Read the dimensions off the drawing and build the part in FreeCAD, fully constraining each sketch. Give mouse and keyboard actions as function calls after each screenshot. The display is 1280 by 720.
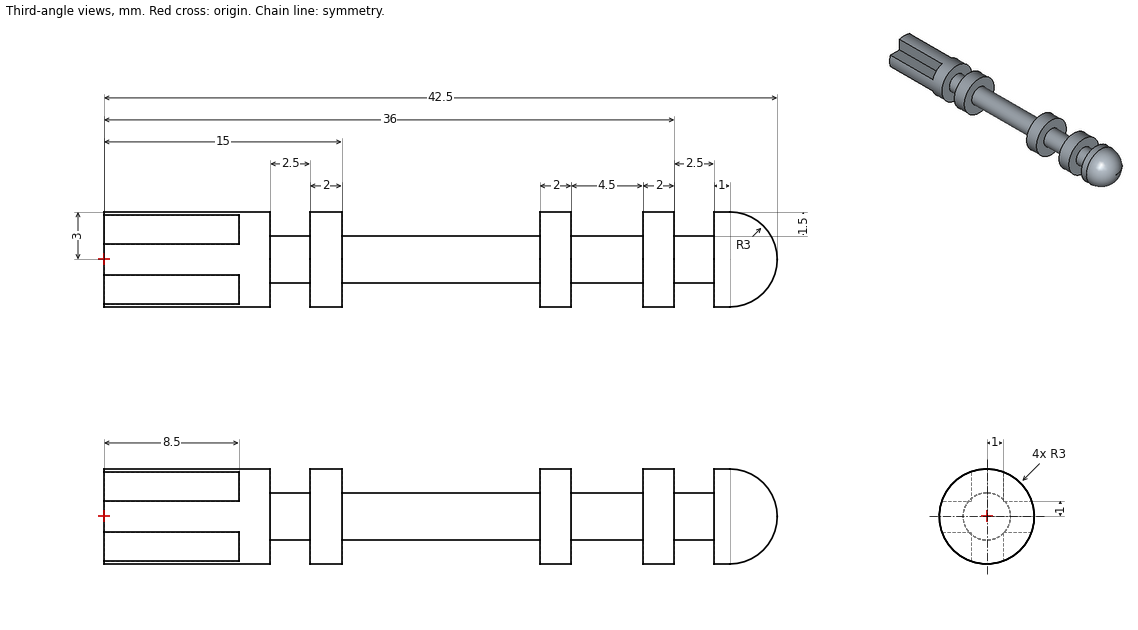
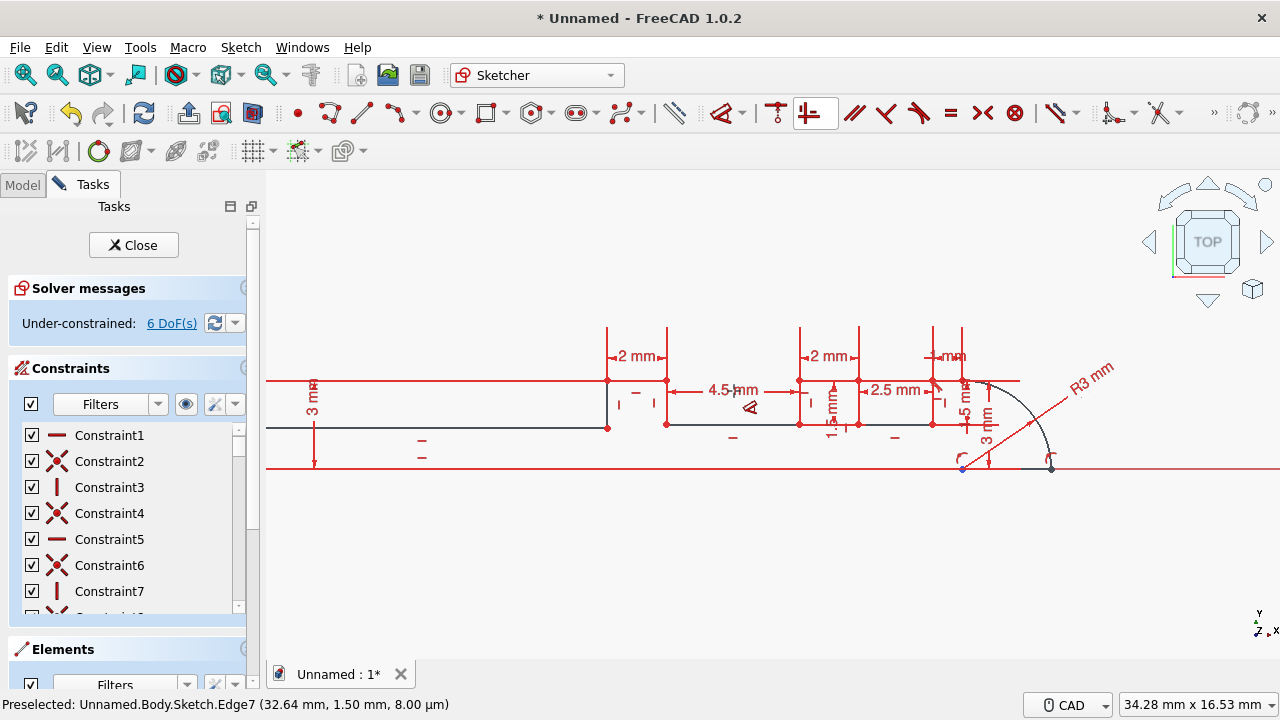
click(607, 395)
click(641, 404)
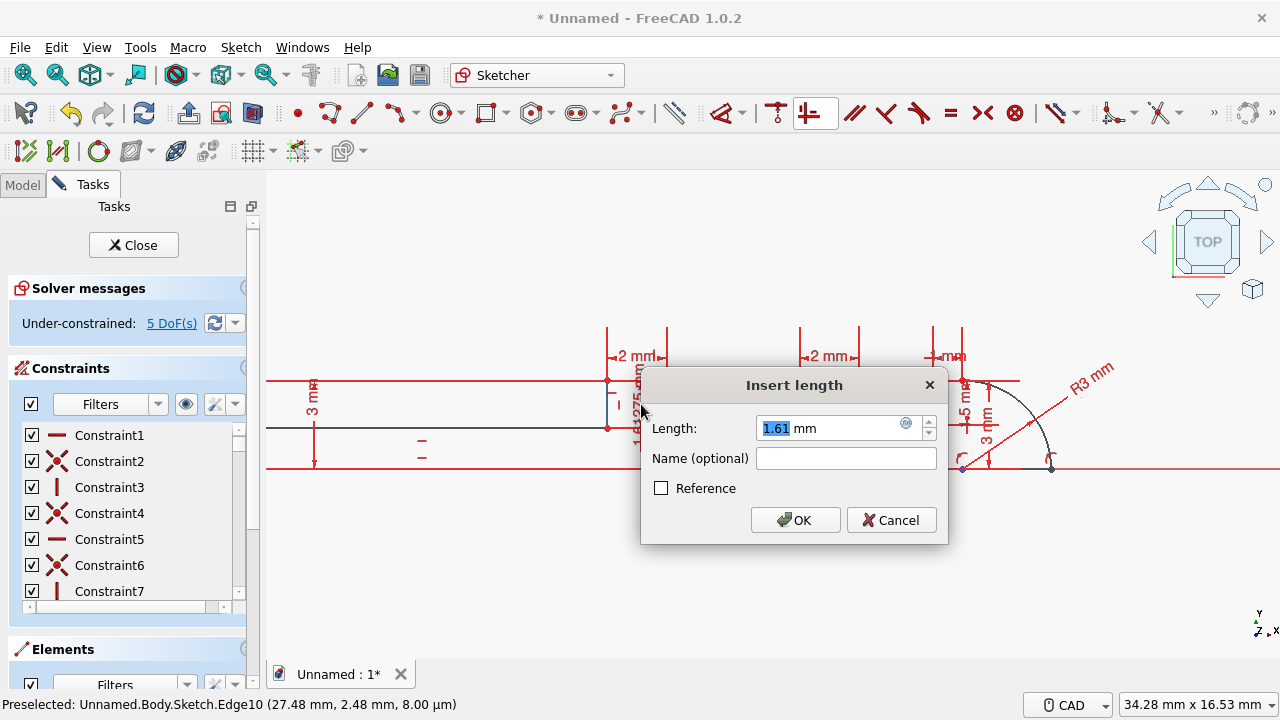
text(1.5)
key(Return)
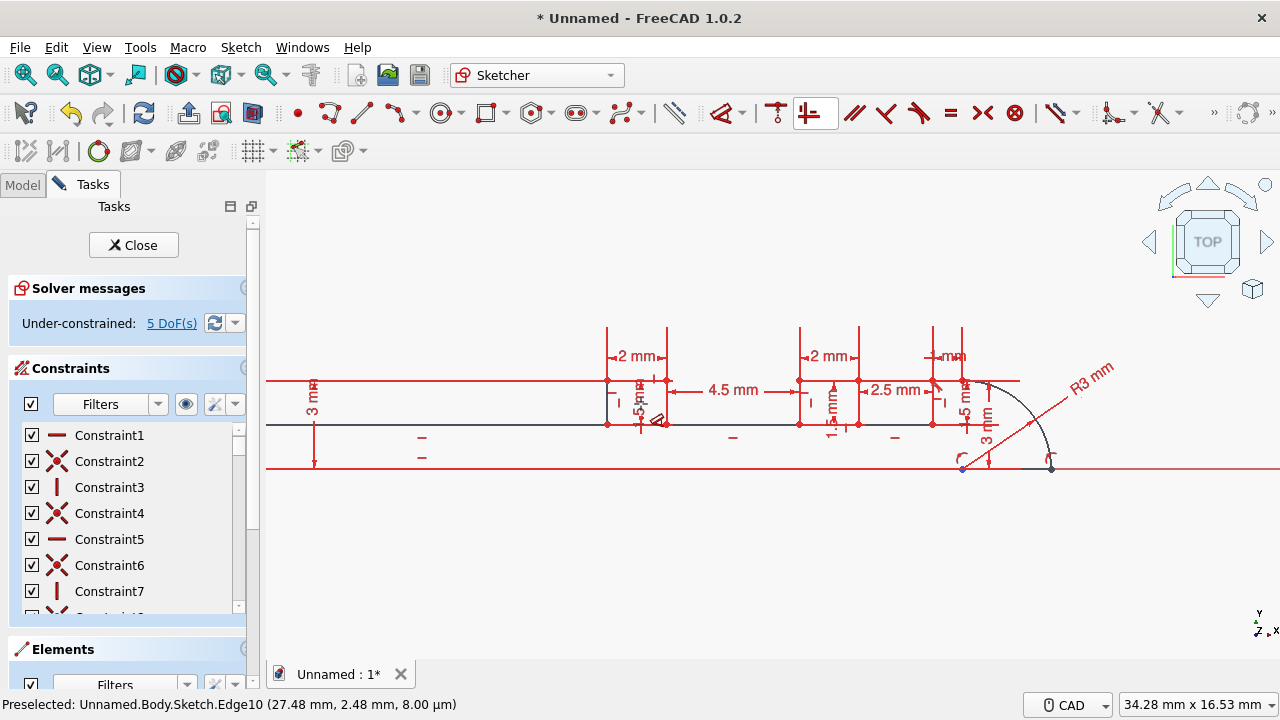
scroll(934, 406, down, 4)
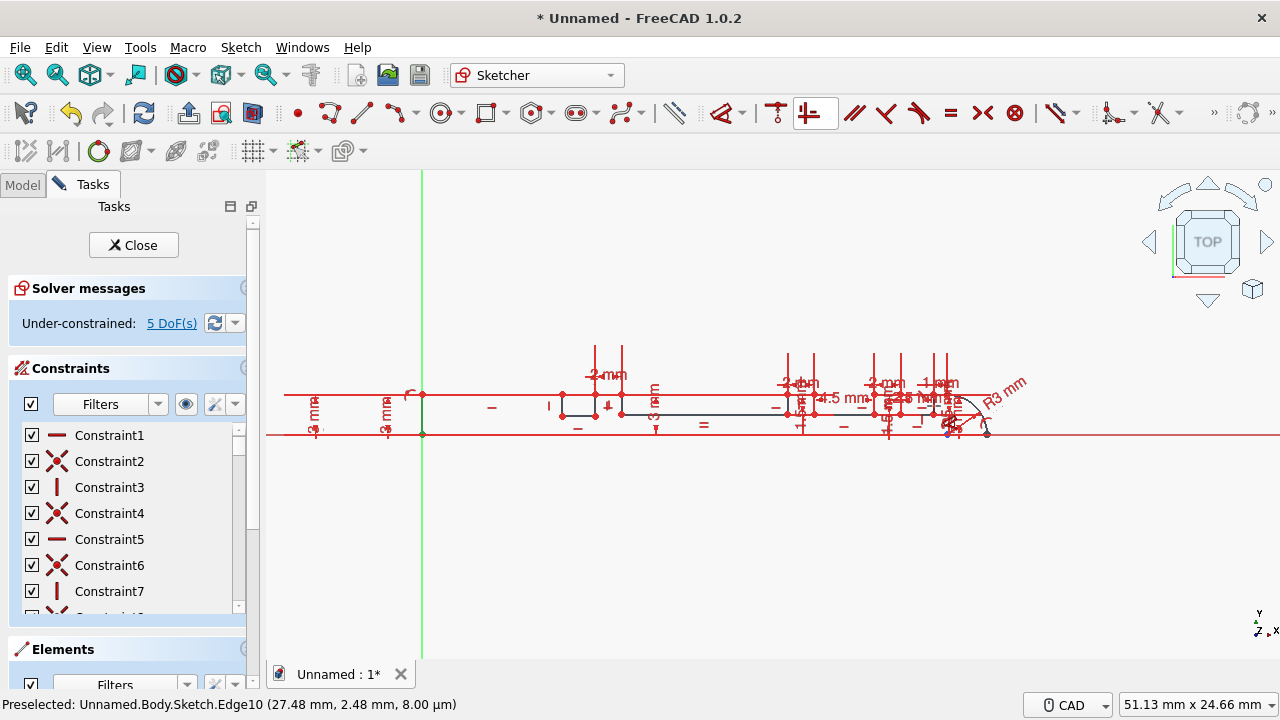
scroll(595, 401, up, 4)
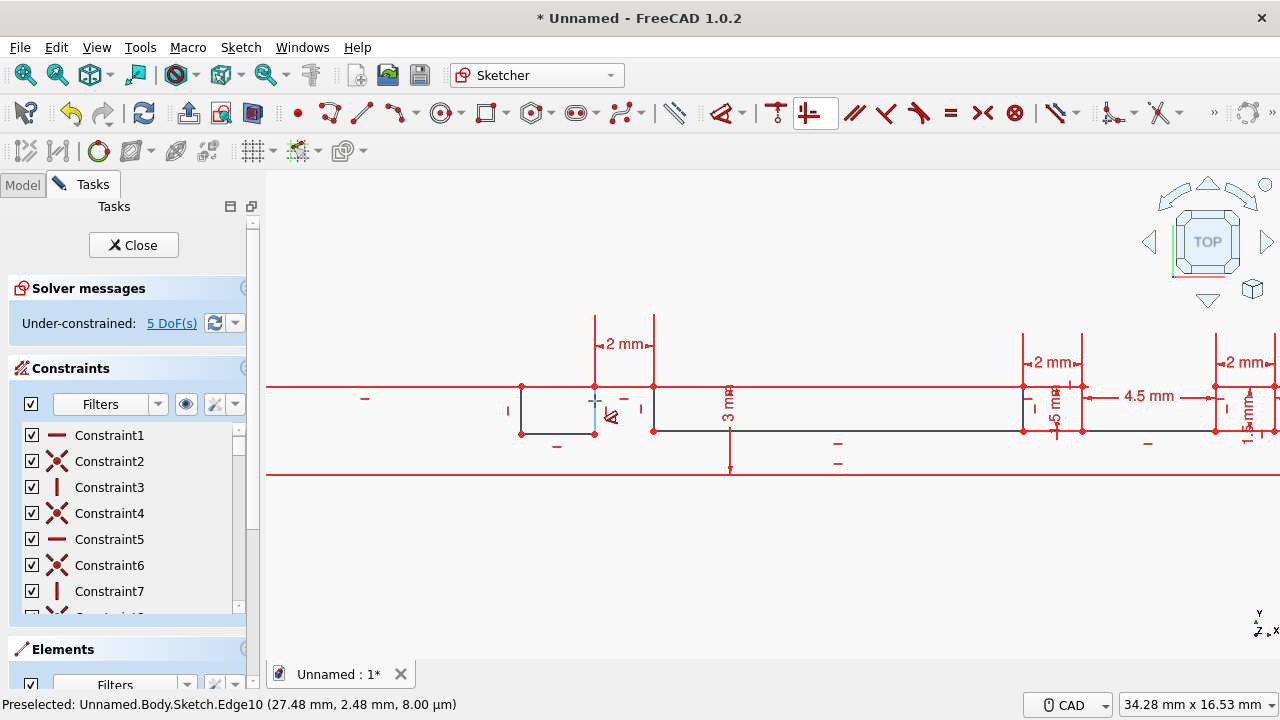
click(595, 401)
click(561, 411)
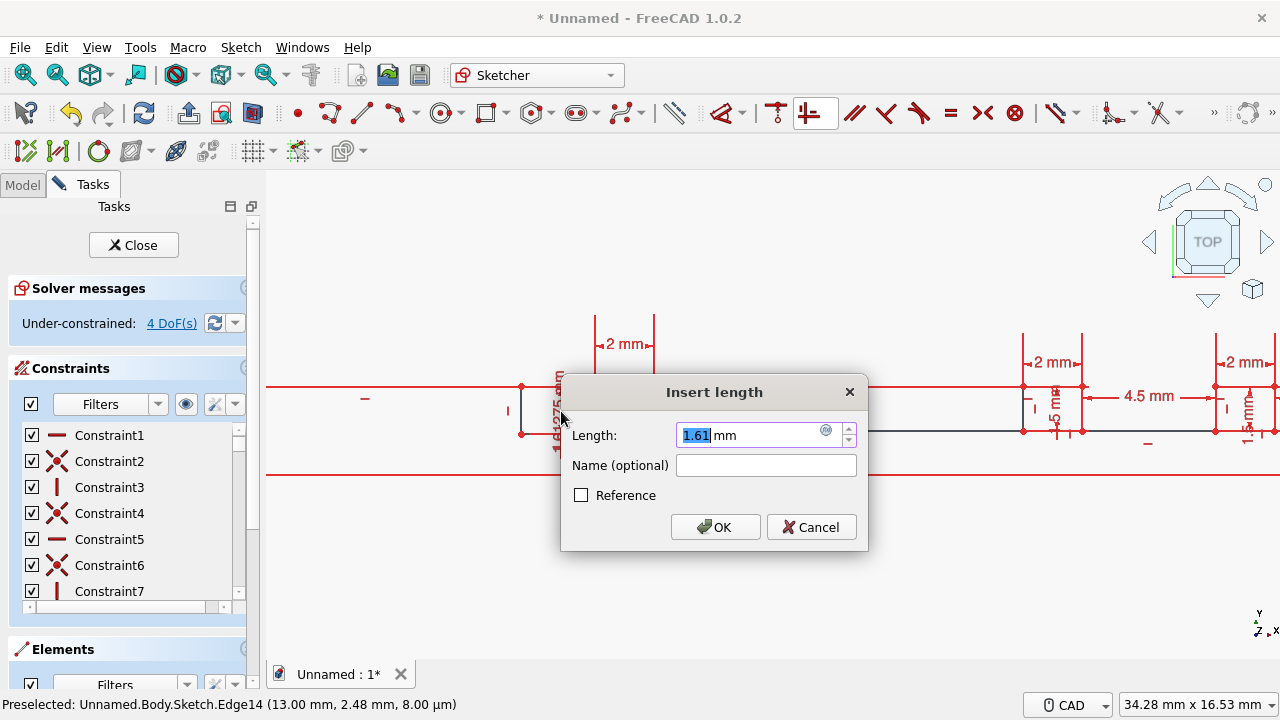
text(1.5)
key(Return)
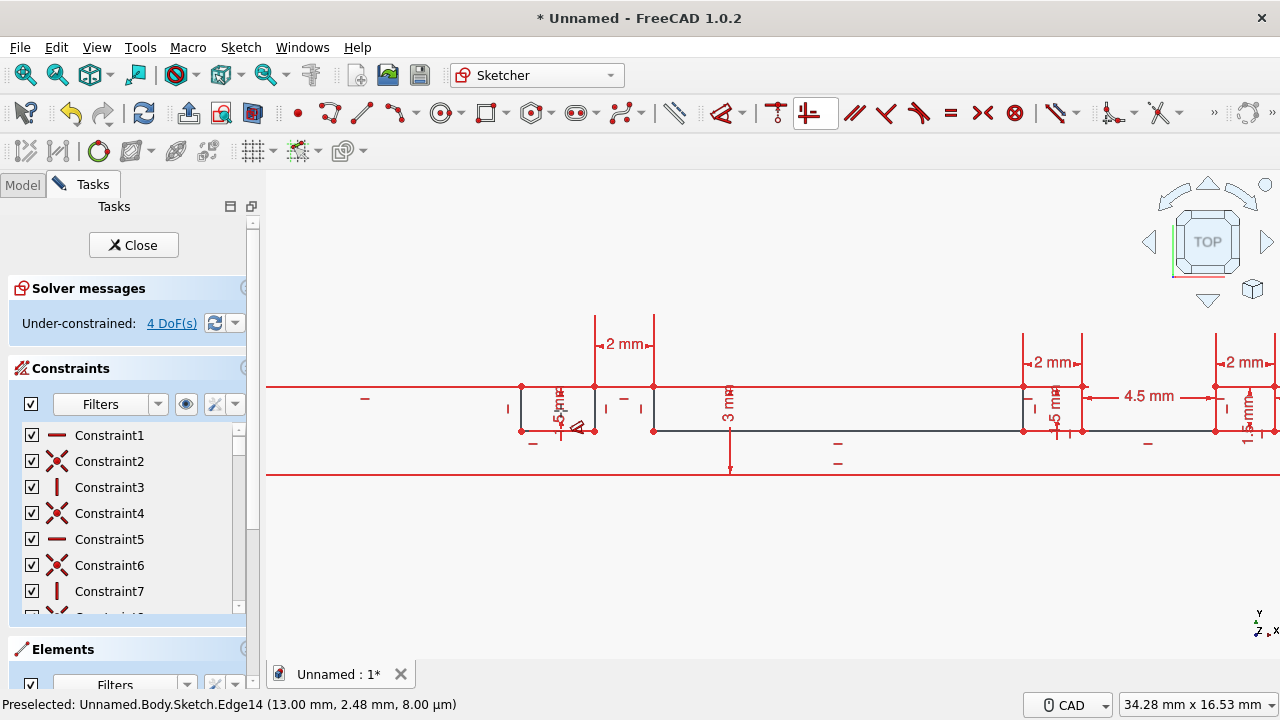
click(573, 431)
click(558, 489)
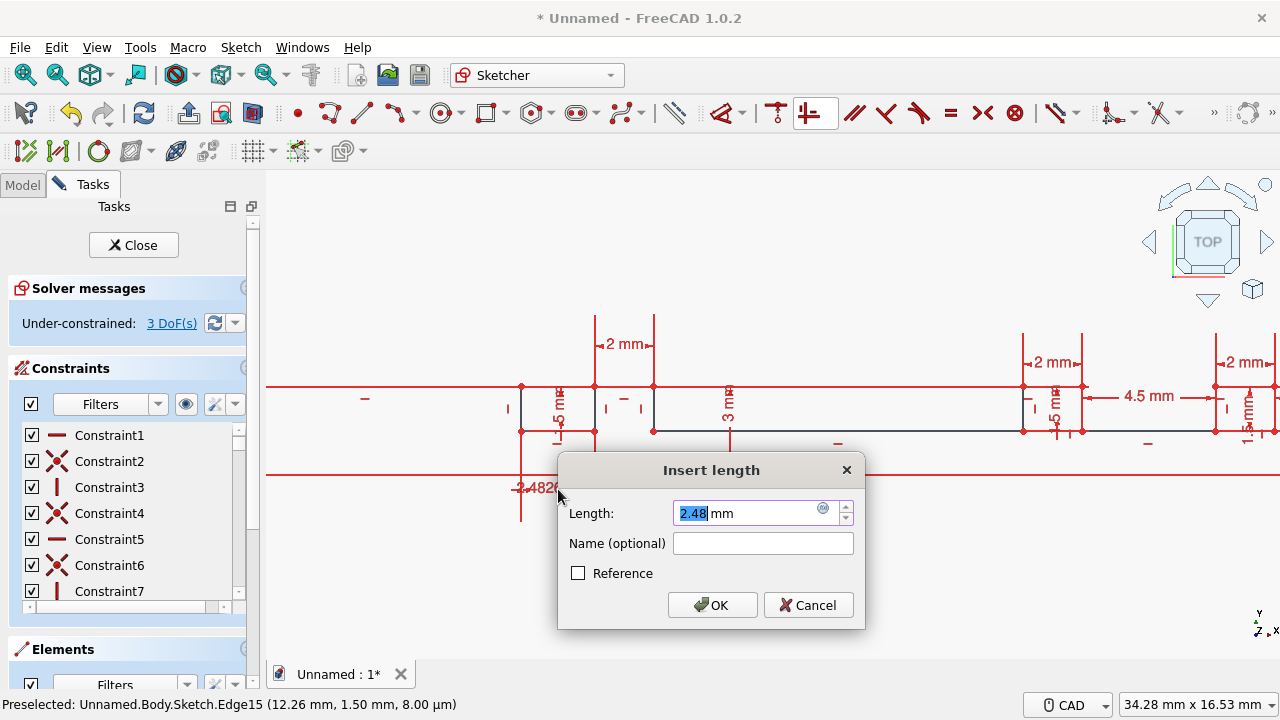
text(2.5)
key(Return)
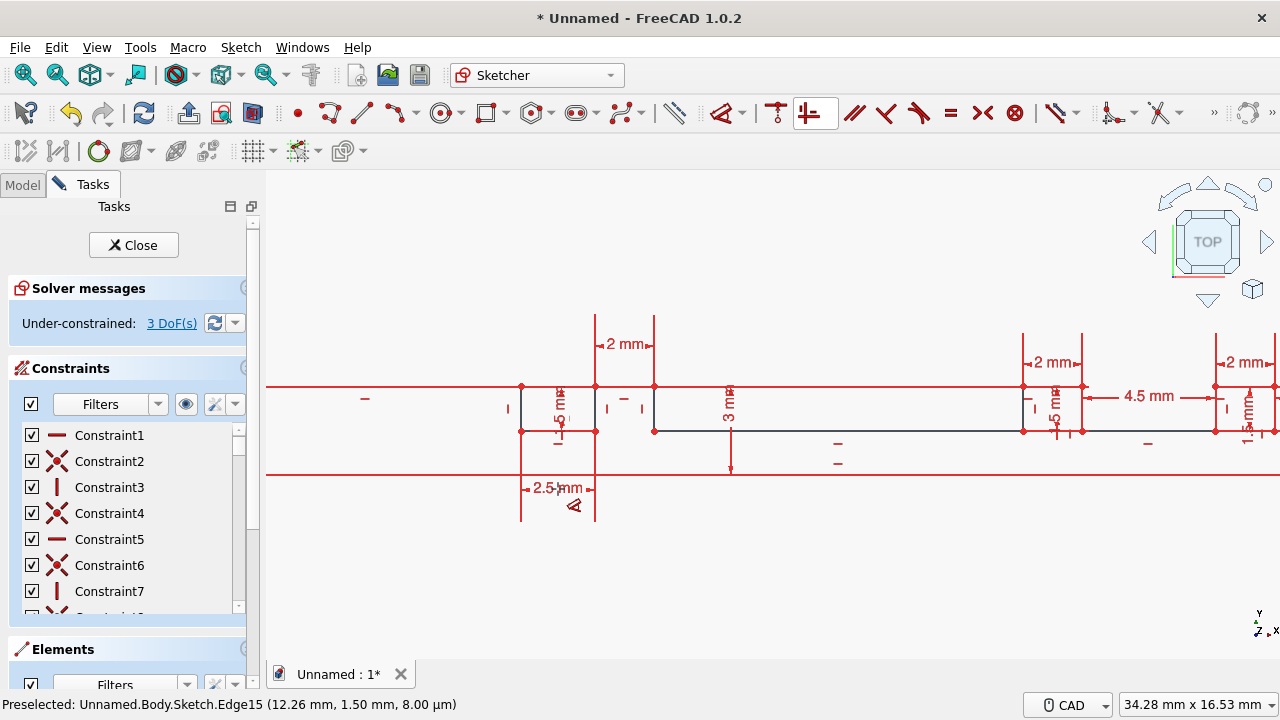
scroll(595, 401, down, 4)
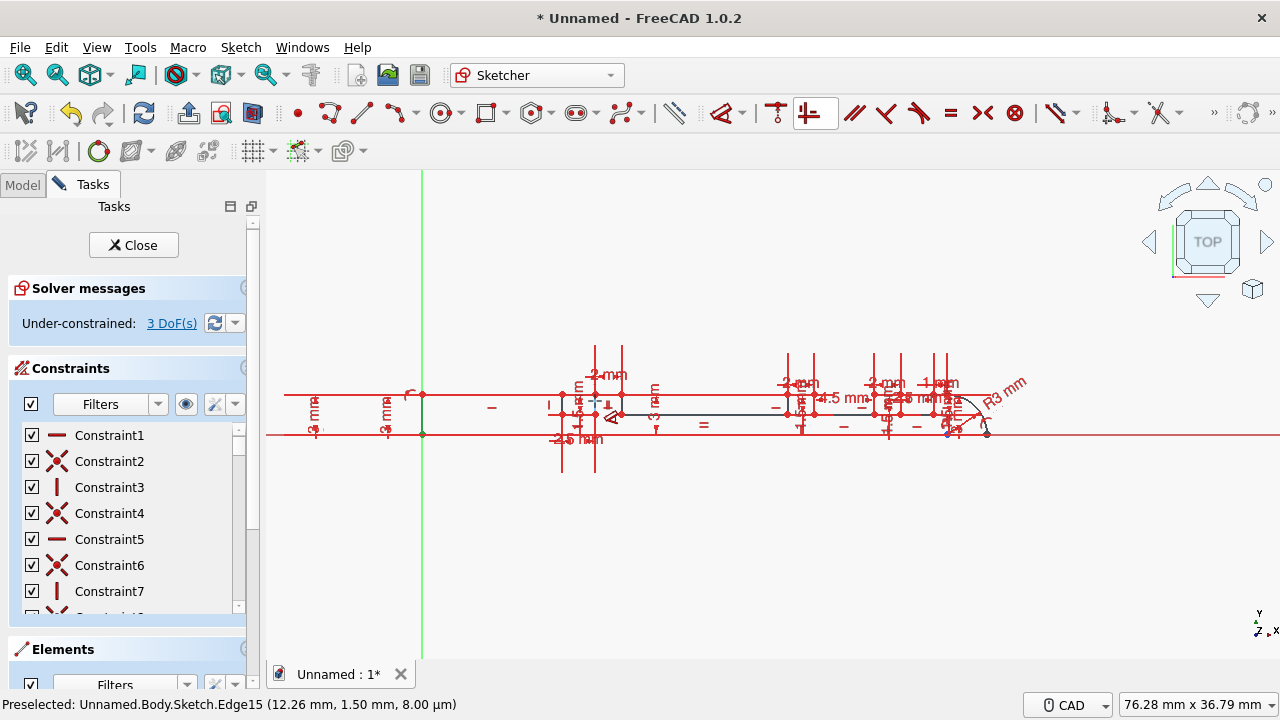
click(901, 415)
click(661, 469)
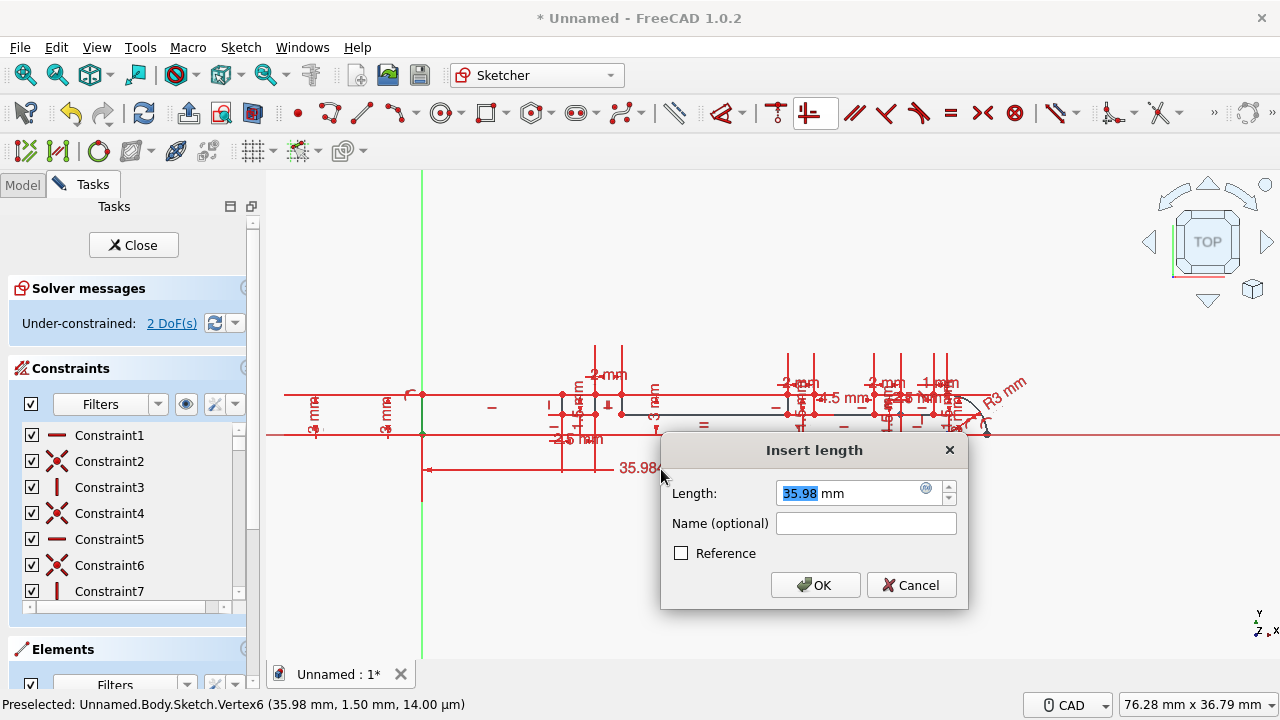
text(36)
key(Return)